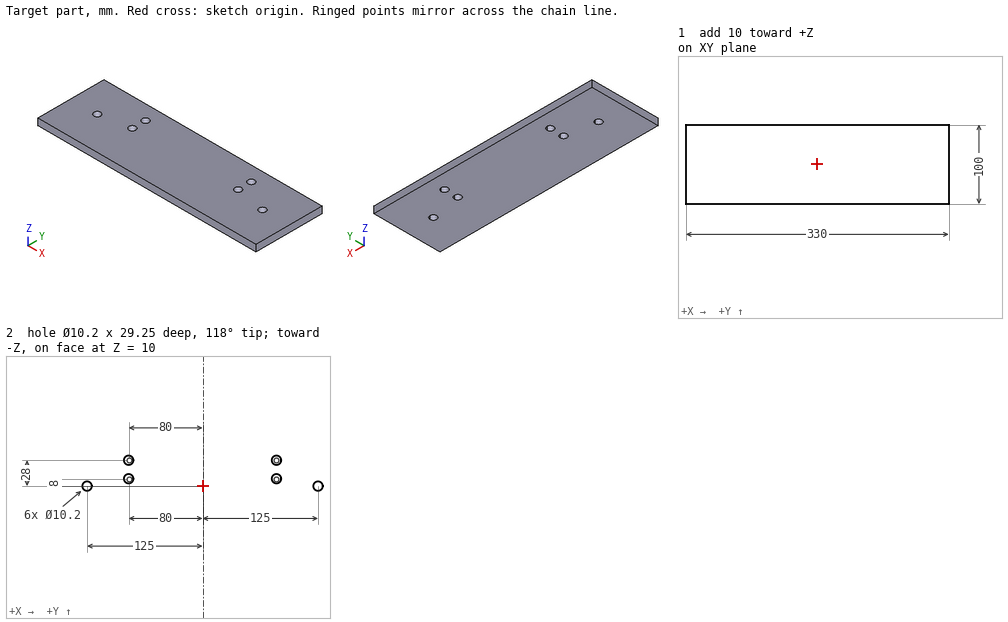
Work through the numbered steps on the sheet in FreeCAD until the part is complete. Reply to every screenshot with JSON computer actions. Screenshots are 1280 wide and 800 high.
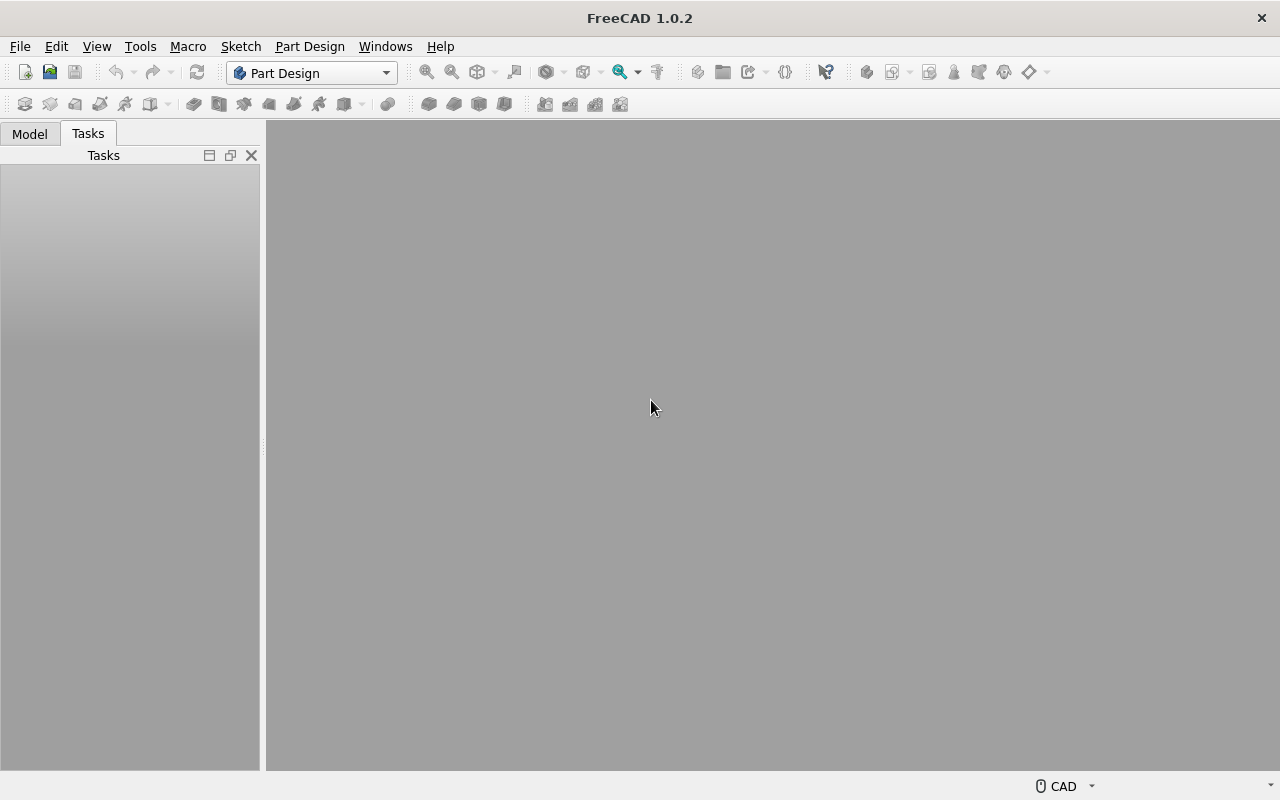
{"action": "left_click", "coordinate": [25, 72]}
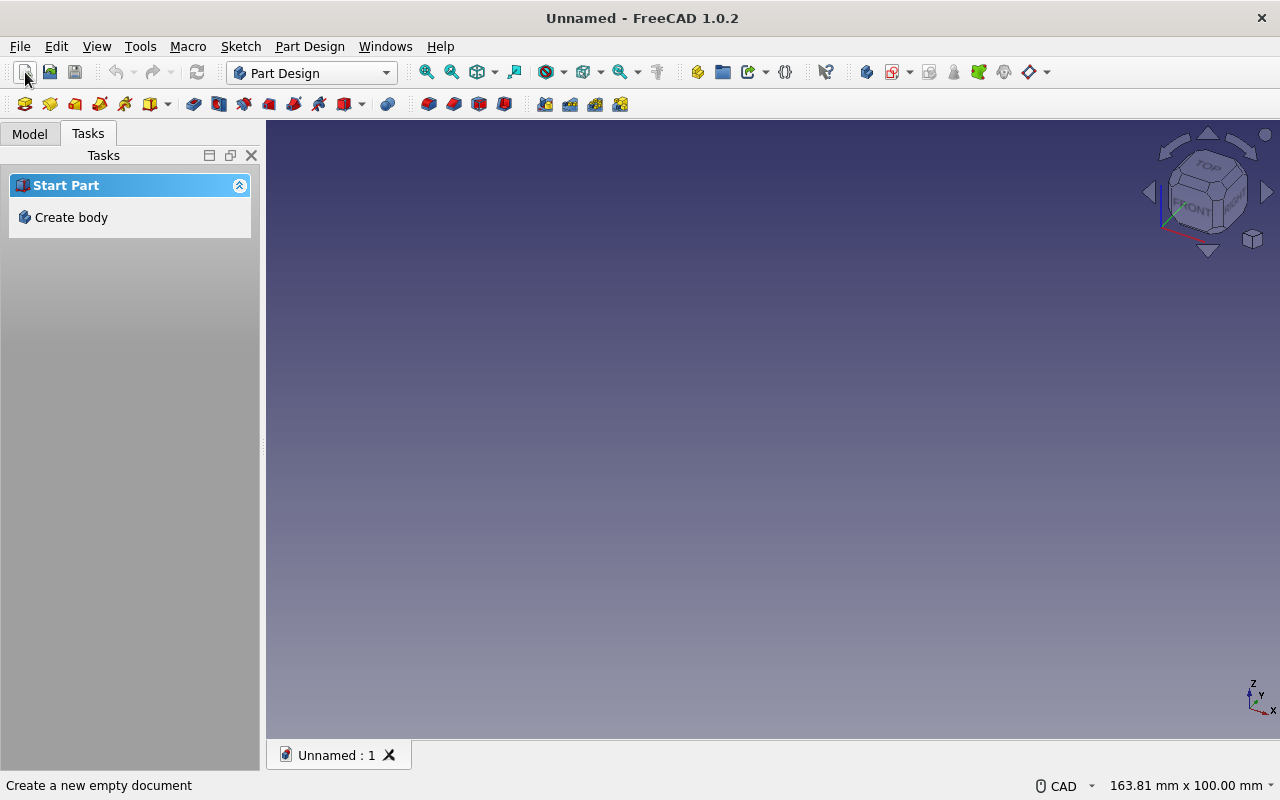
{"action": "left_click", "coordinate": [892, 72]}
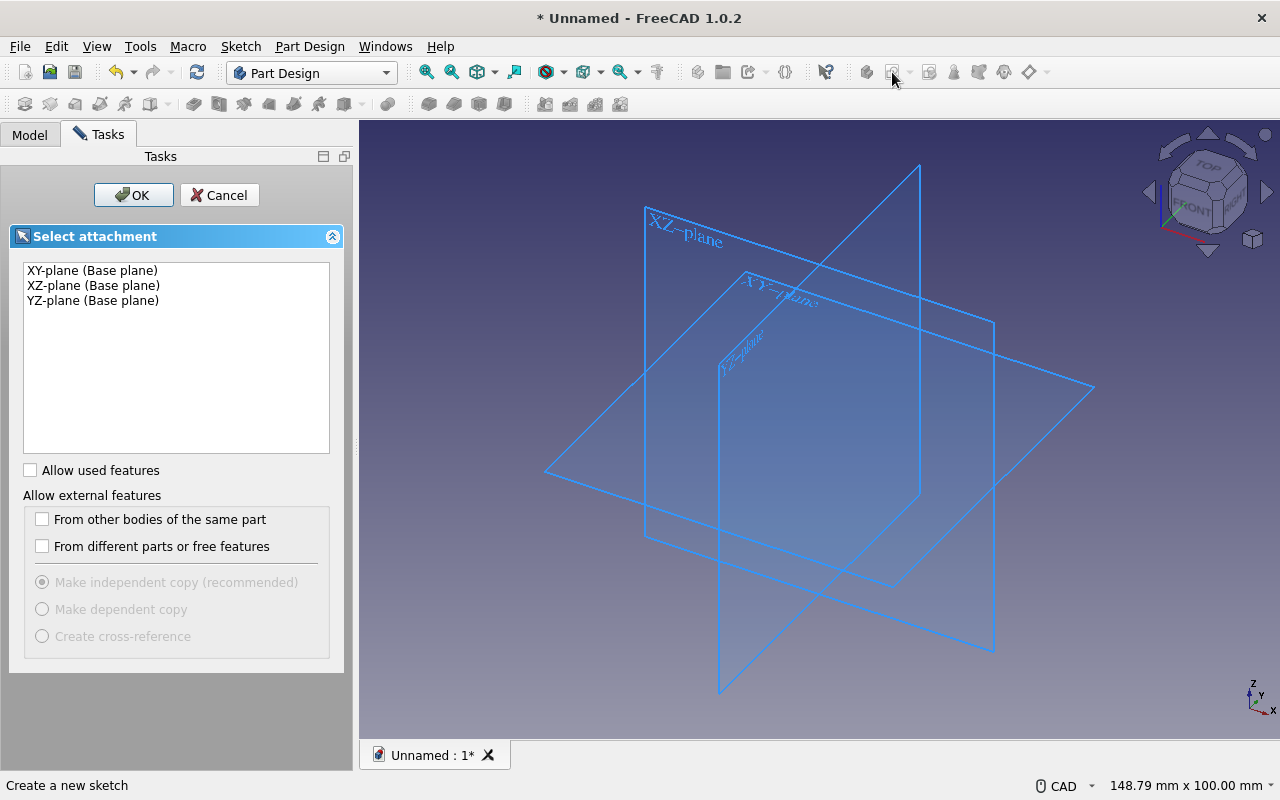
{"action": "left_click", "coordinate": [84, 270]}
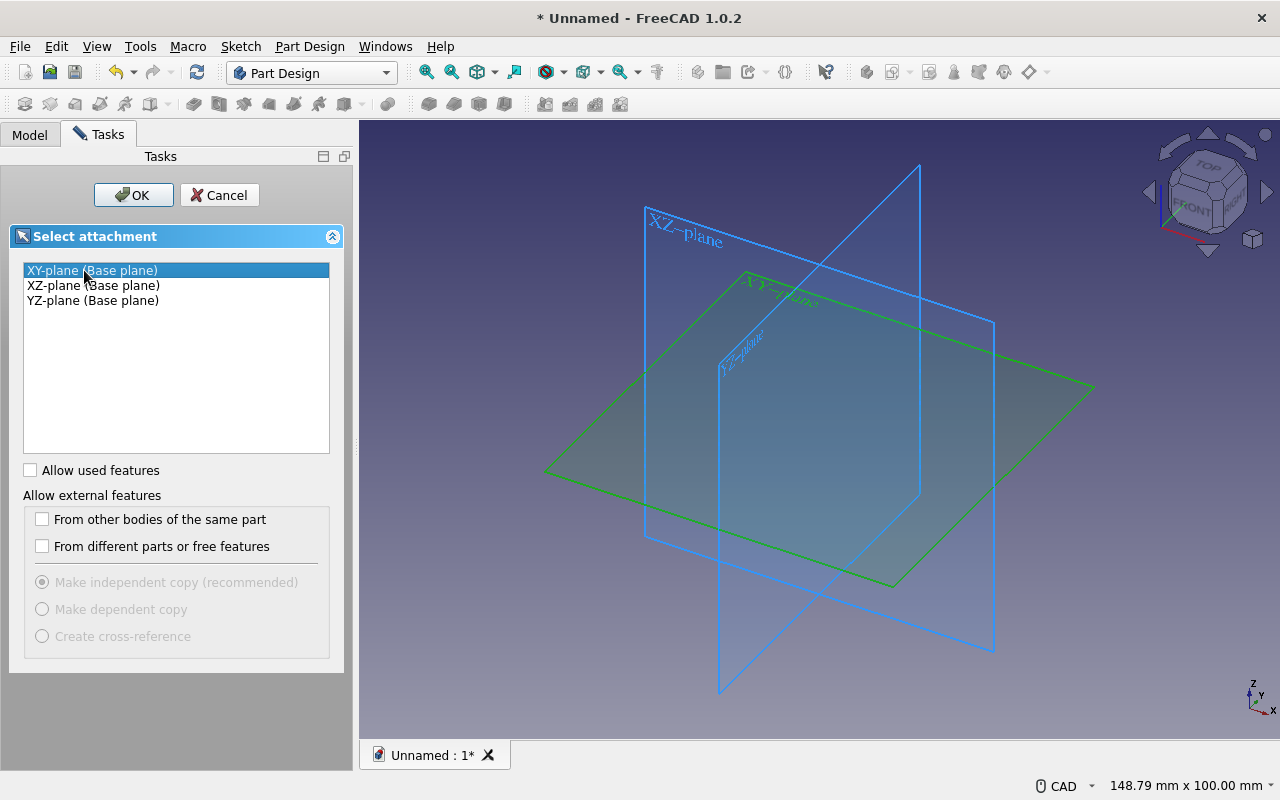
{"action": "left_click", "coordinate": [134, 195]}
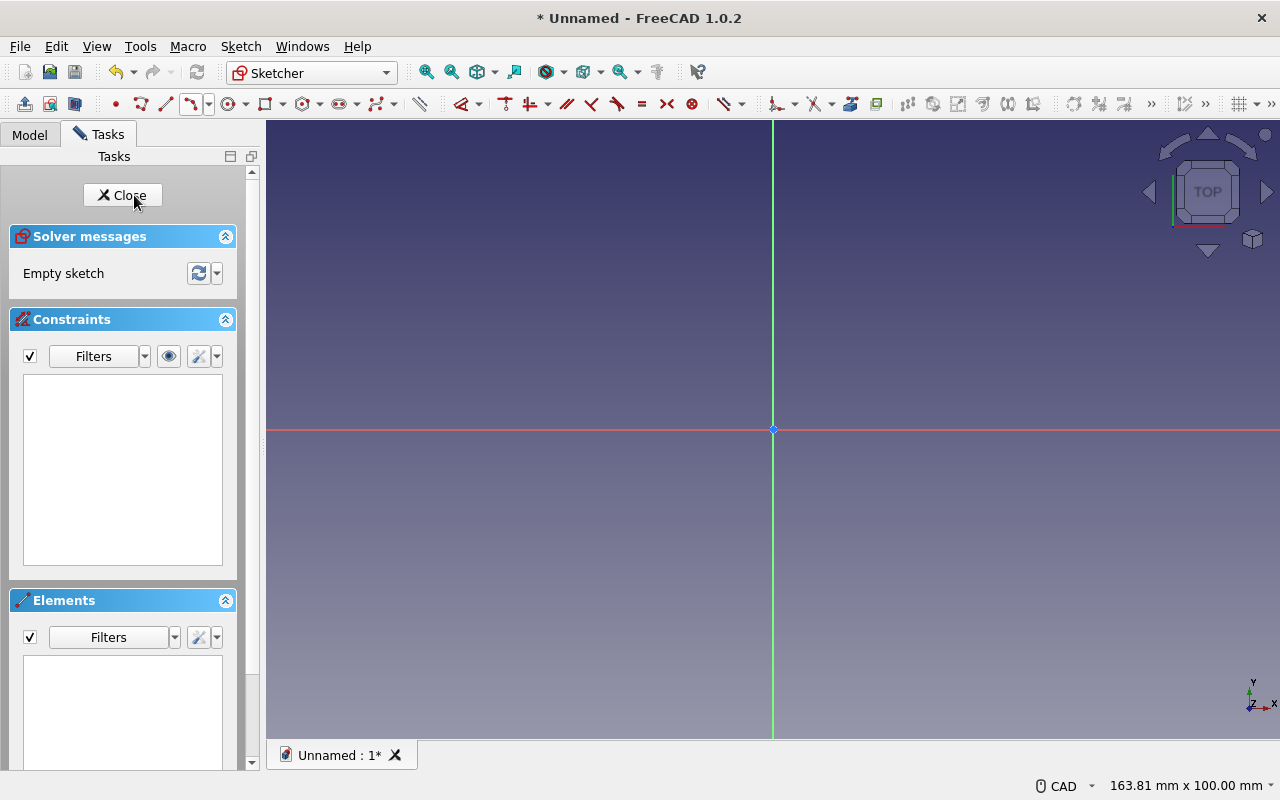
{"action": "scroll", "coordinate": [675, 429], "scroll_direction": "down", "scroll_amount": 6}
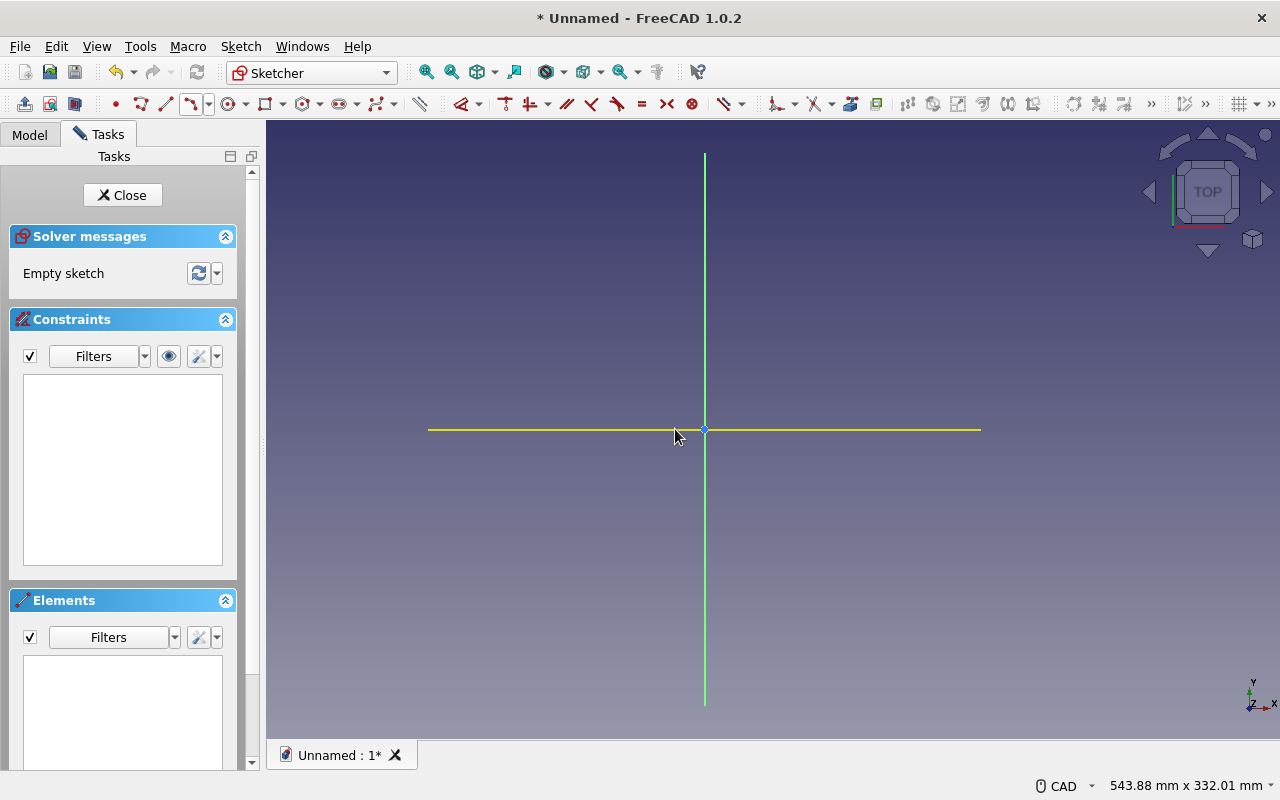
{"action": "left_click", "coordinate": [282, 104]}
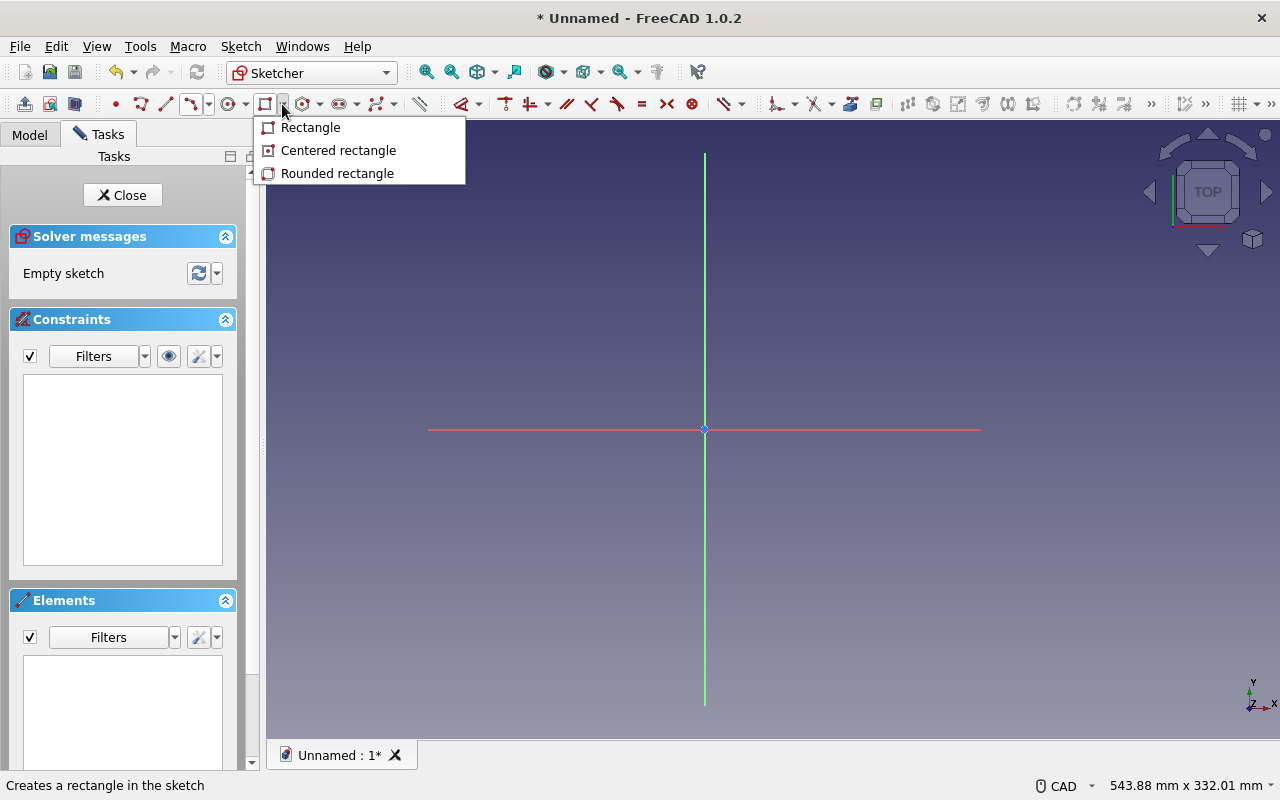
{"action": "left_click", "coordinate": [360, 150]}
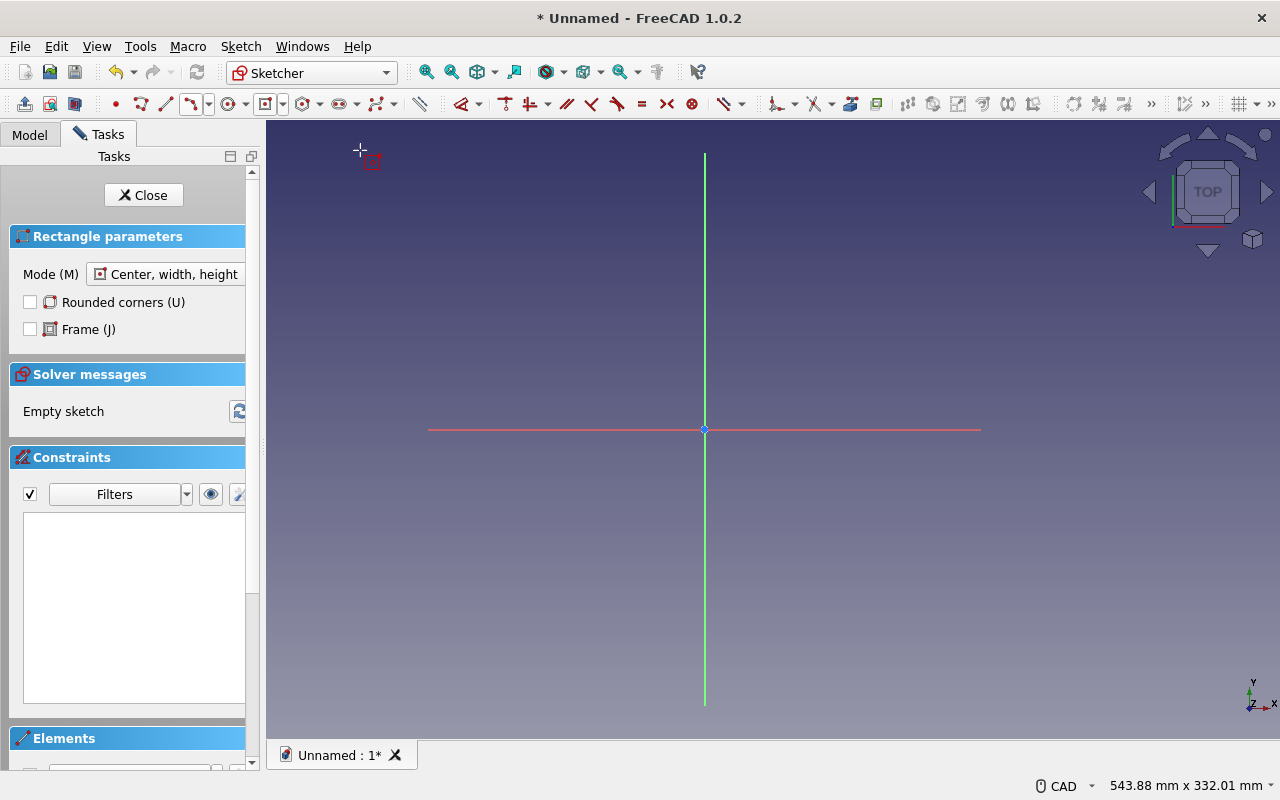
{"action": "left_click", "coordinate": [705, 430]}
{"action": "mouse_move", "coordinate": [1012, 336]}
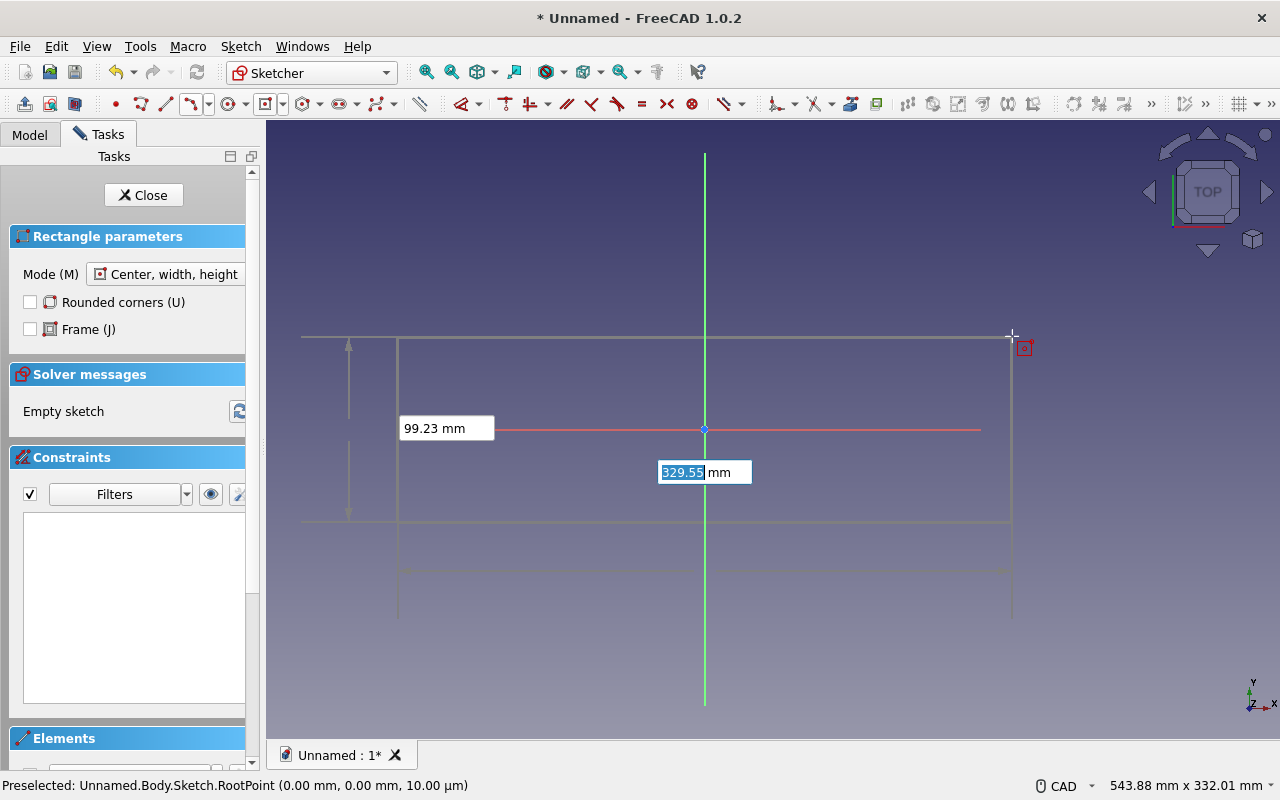
{"action": "type", "text": "330"}
{"action": "key", "text": "Tab"}
{"action": "type", "text": "100"}
{"action": "key", "text": "Return"}
{"action": "key", "text": "Escape"}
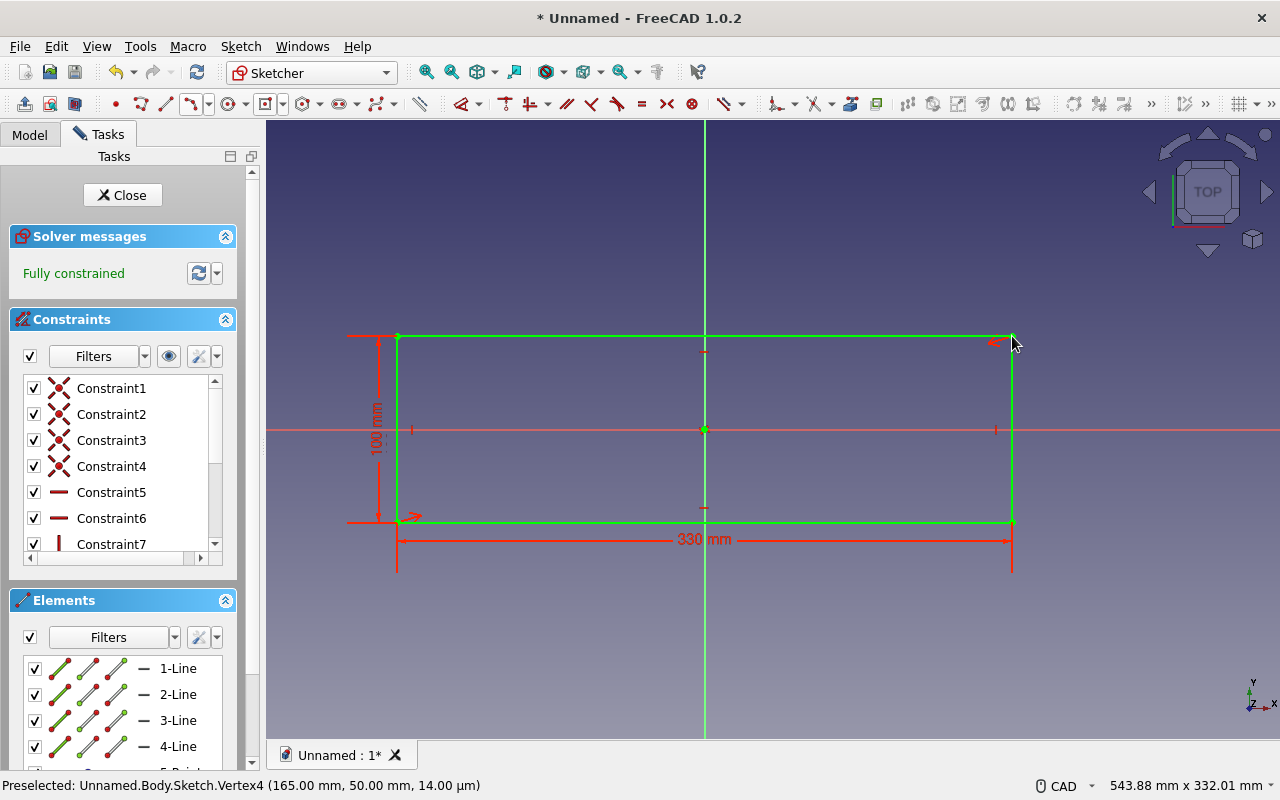
{"action": "left_click", "coordinate": [123, 195]}